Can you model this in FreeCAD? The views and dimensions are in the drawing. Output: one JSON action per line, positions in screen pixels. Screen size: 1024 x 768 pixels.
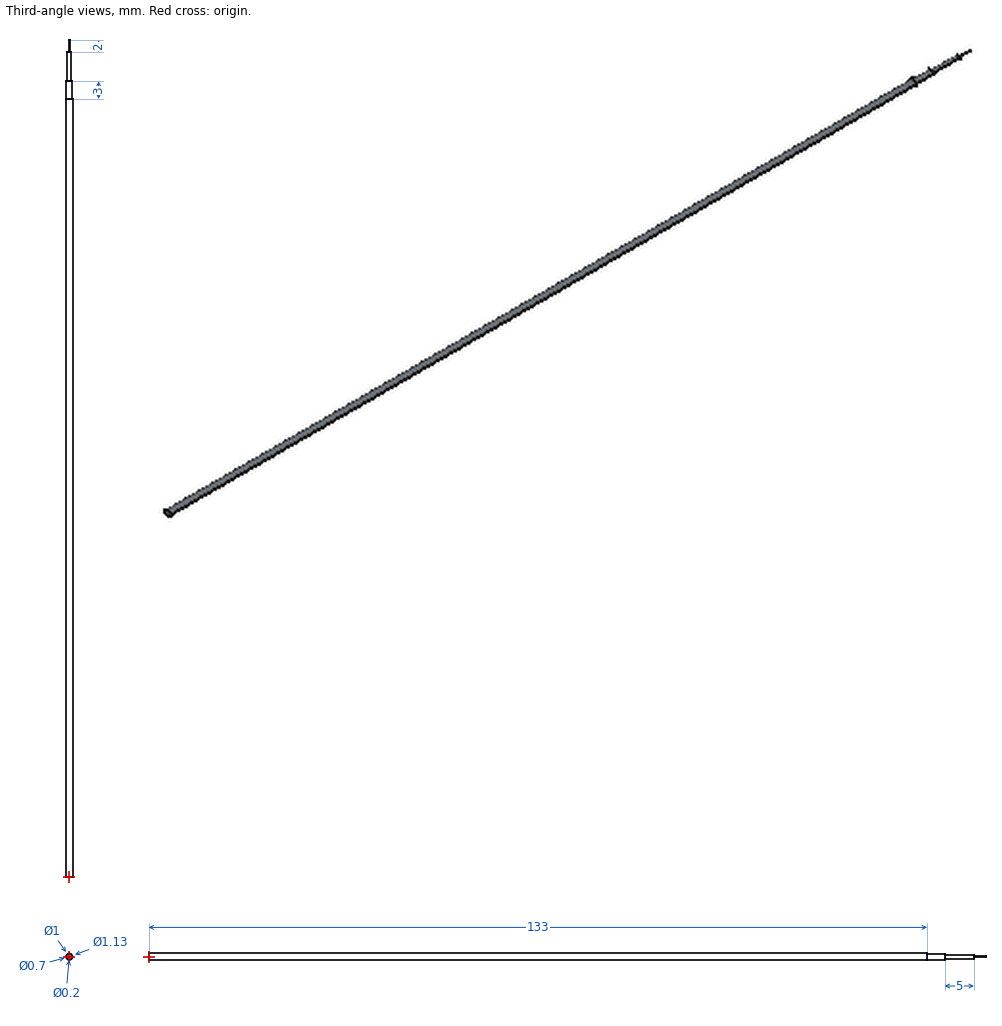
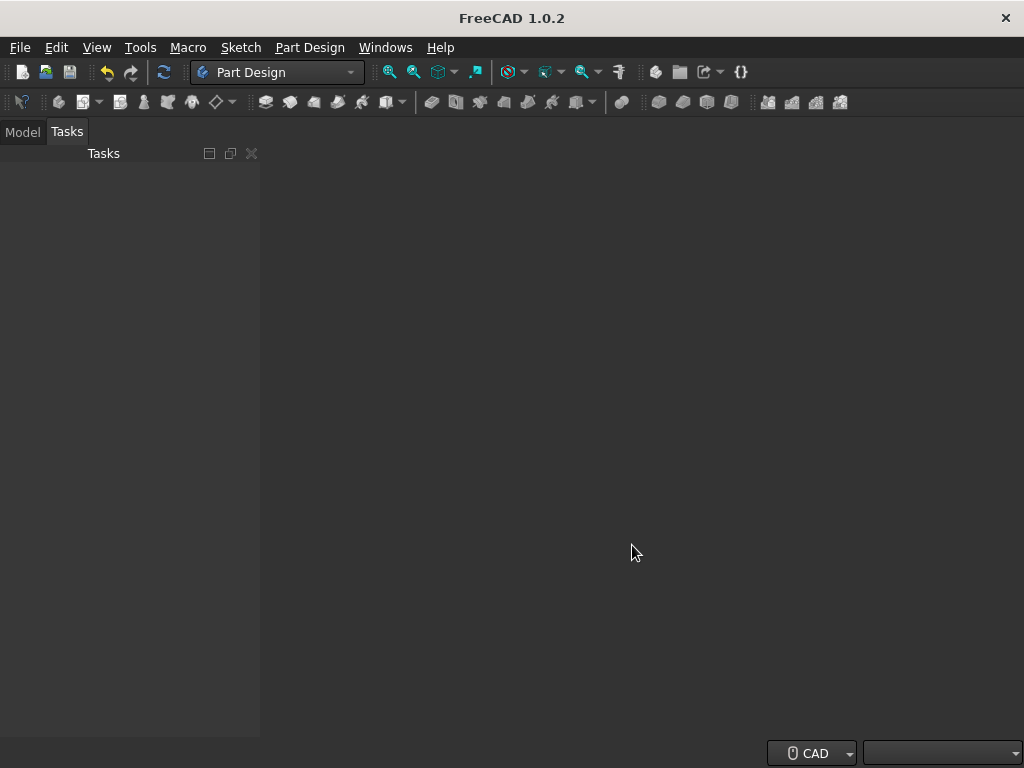
{"action": "left_click", "coordinate": [22, 72]}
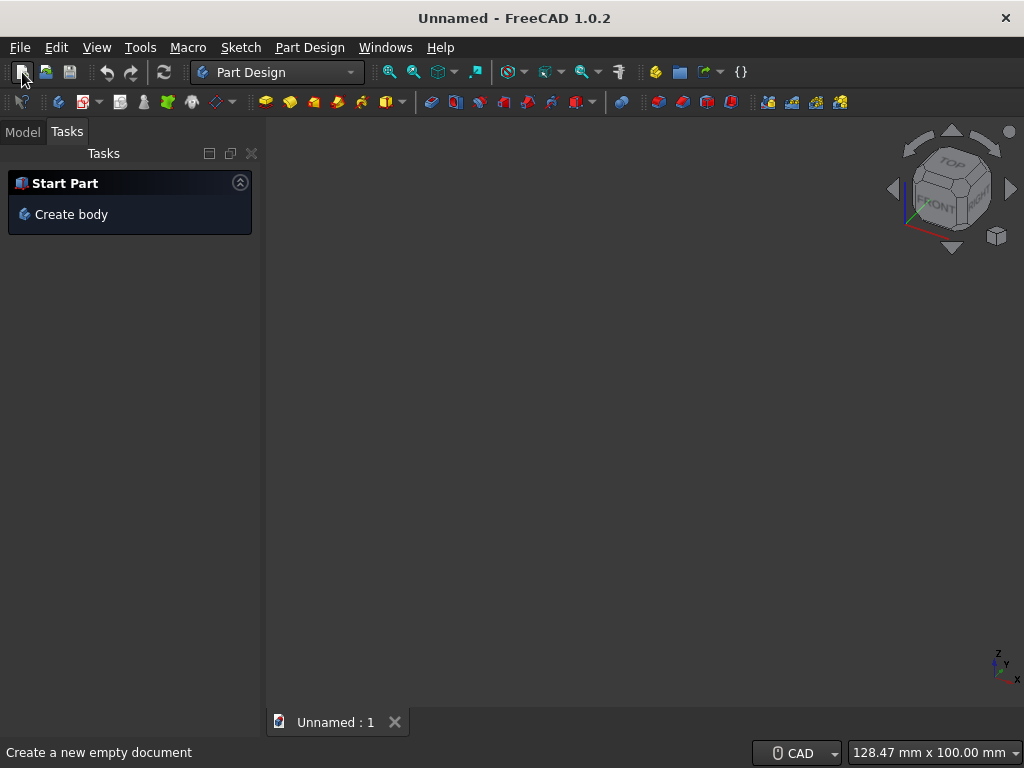
{"action": "left_click", "coordinate": [84, 102]}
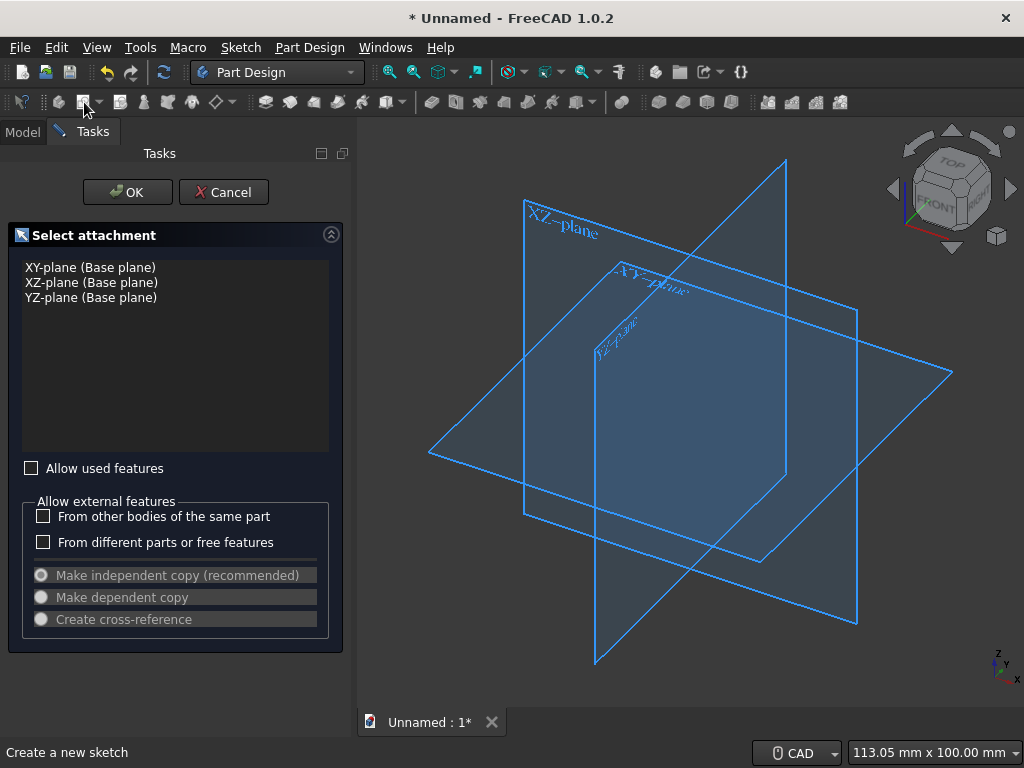
{"action": "left_click", "coordinate": [82, 282]}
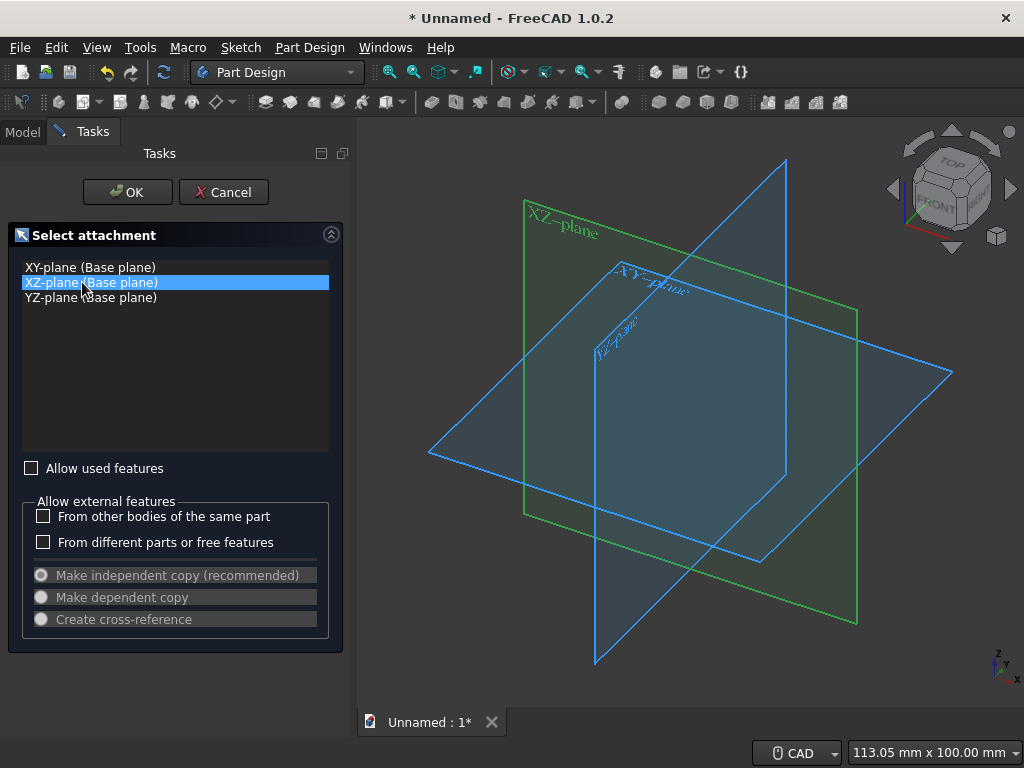
{"action": "left_click", "coordinate": [128, 192]}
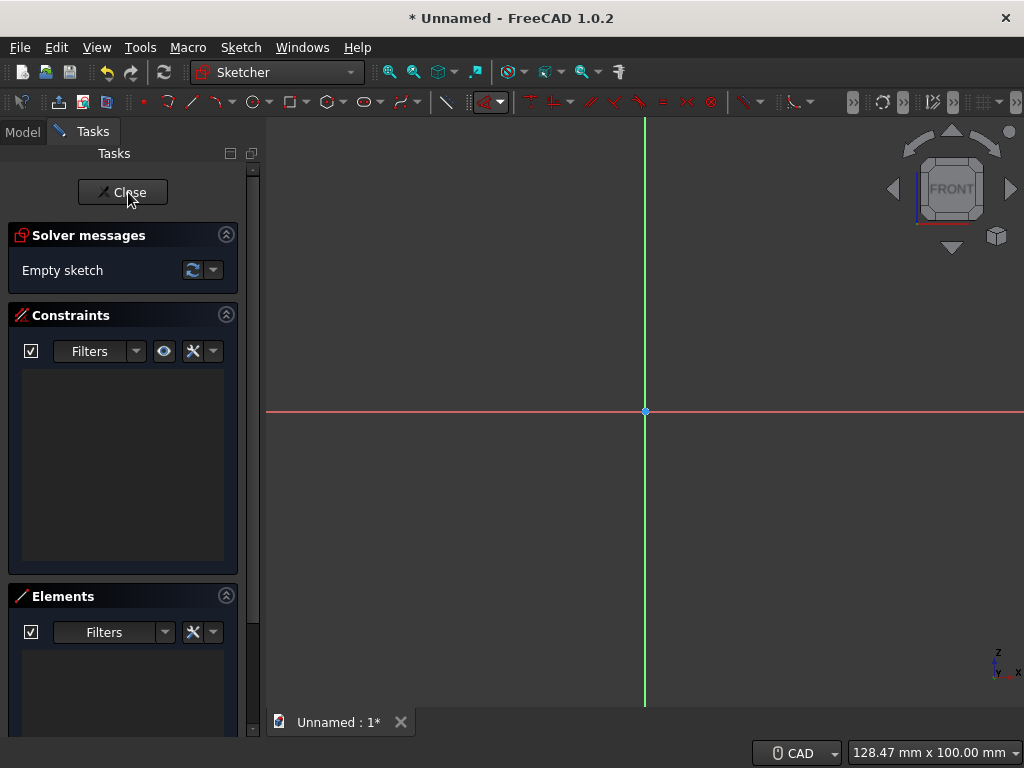
{"action": "scroll", "coordinate": [649, 412], "scroll_direction": "up", "scroll_amount": 15}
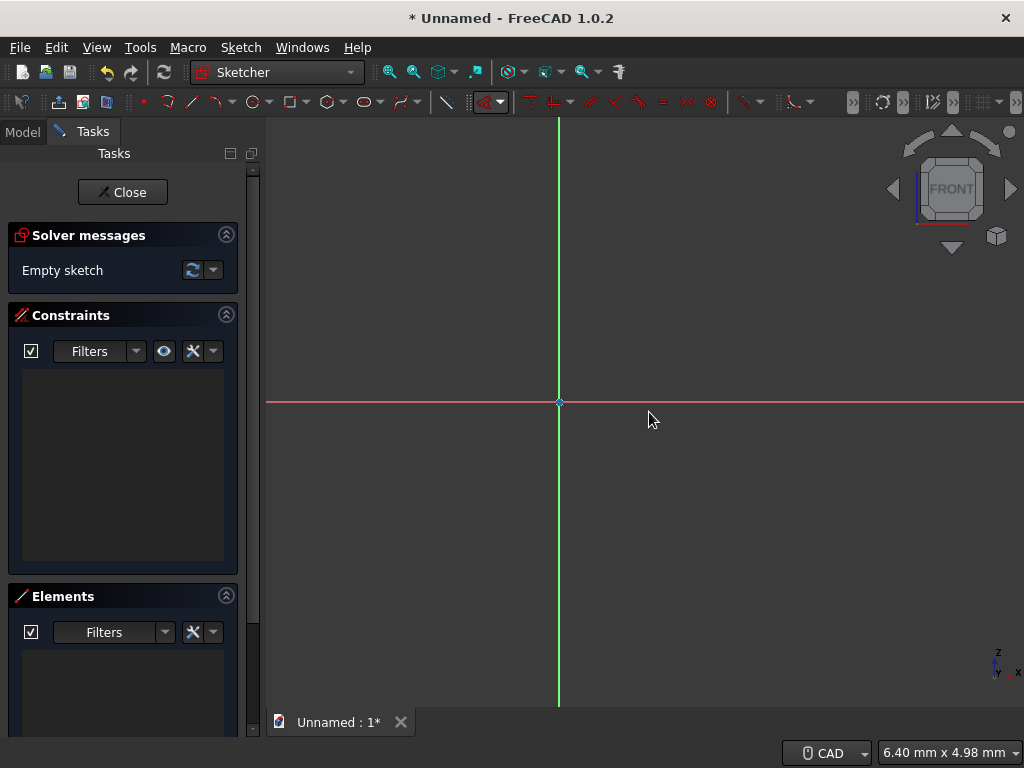
{"action": "scroll", "coordinate": [549, 397], "scroll_direction": "up", "scroll_amount": 5}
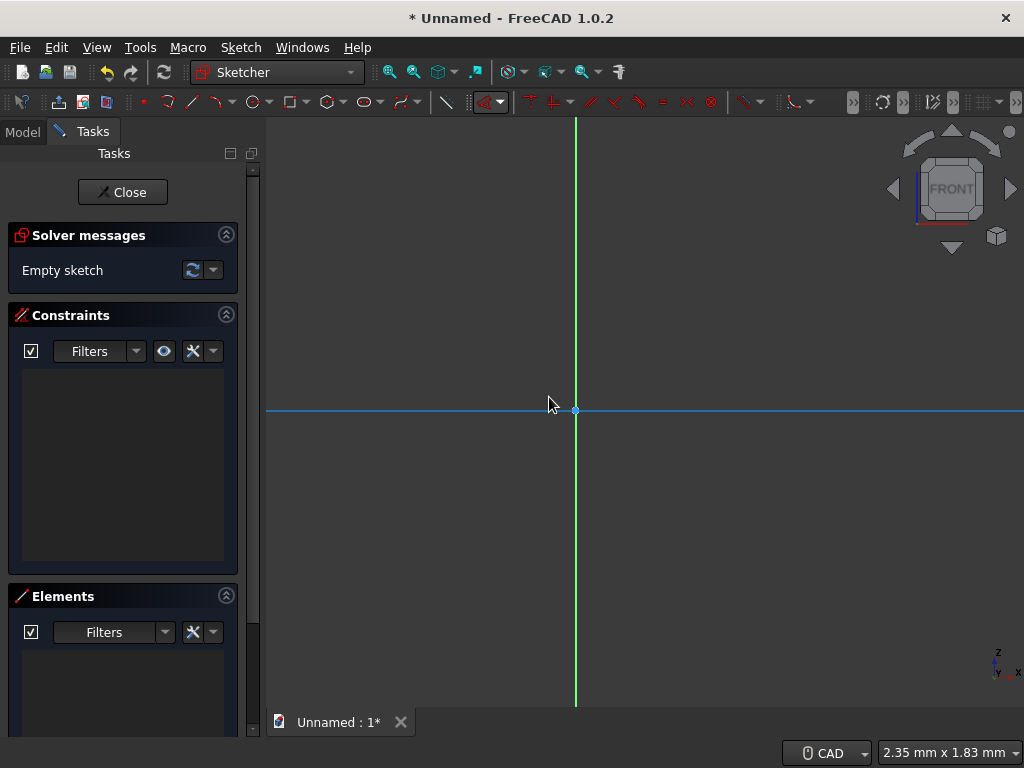
{"action": "left_click", "coordinate": [254, 102]}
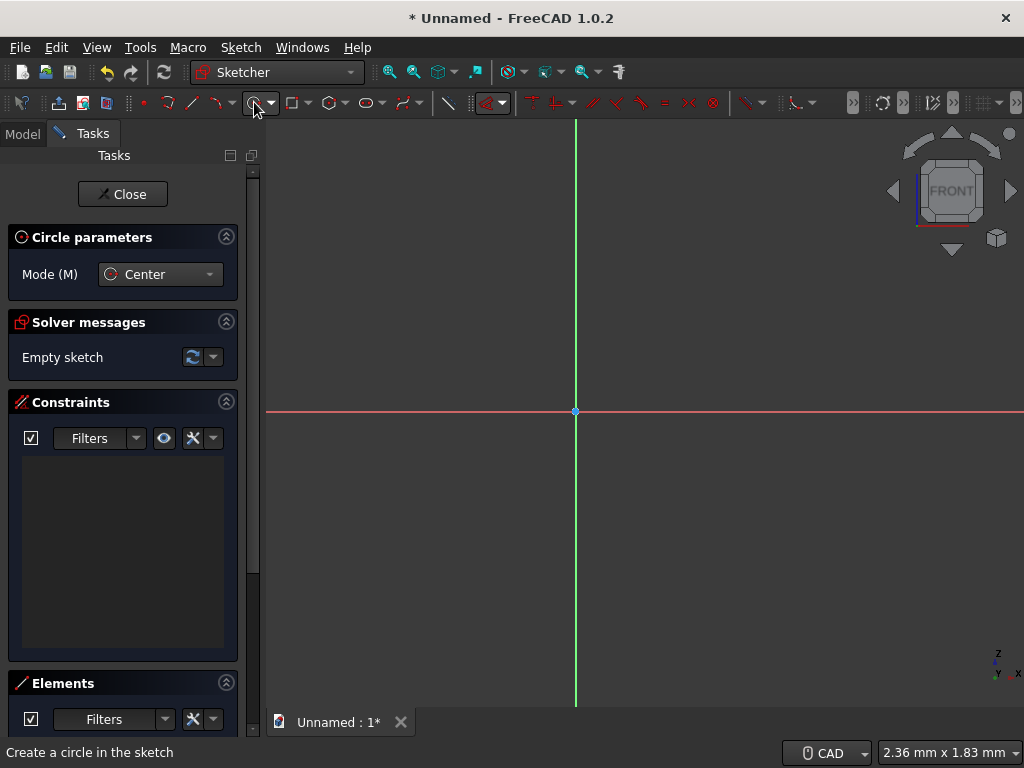
{"action": "left_click", "coordinate": [576, 412]}
{"action": "left_click", "coordinate": [704, 284]}
{"action": "key", "text": "Escape"}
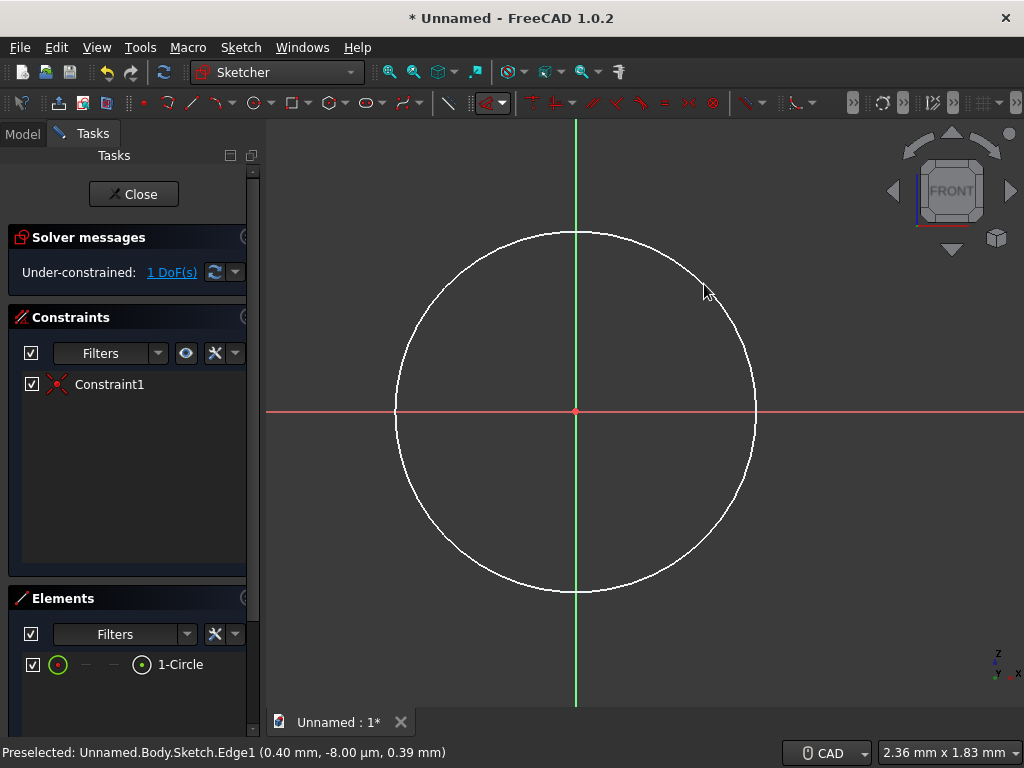
{"action": "left_click", "coordinate": [703, 284]}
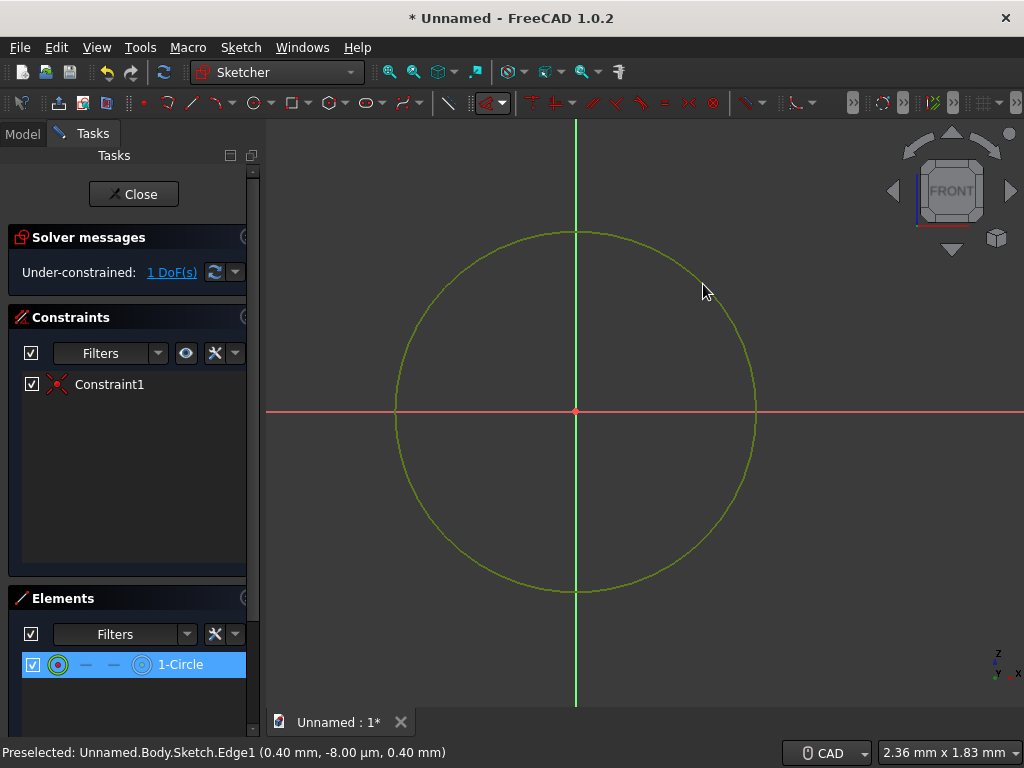
{"action": "key", "text": "k o"}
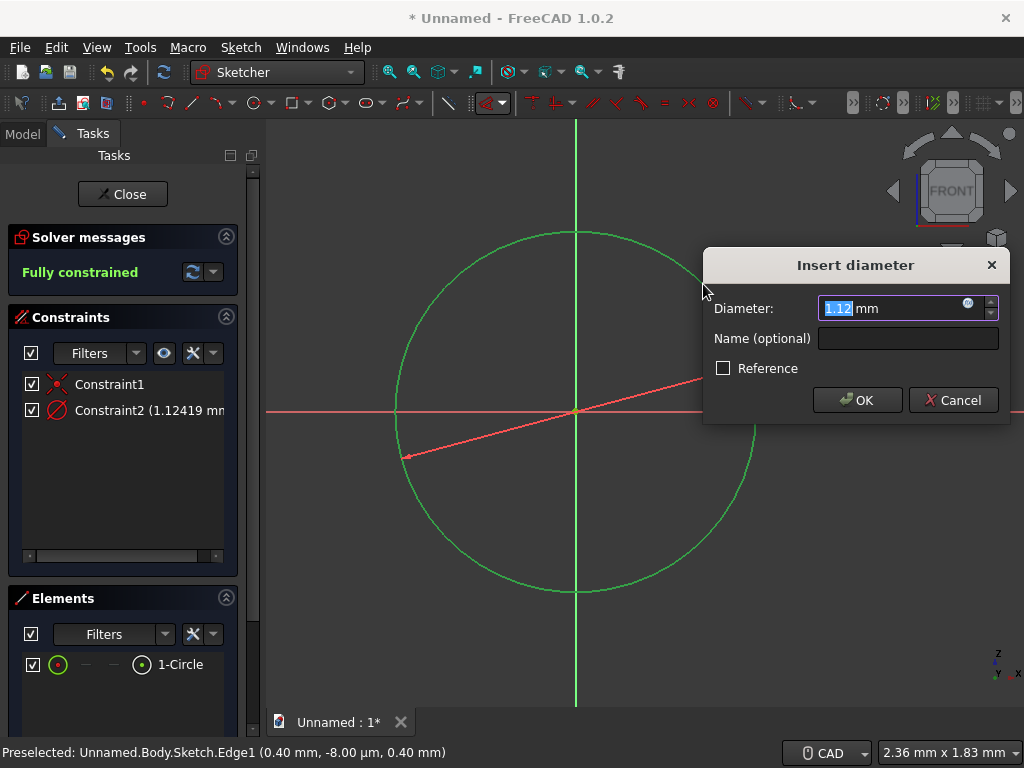
{"action": "type", "text": "1.13"}
{"action": "key", "text": "Return"}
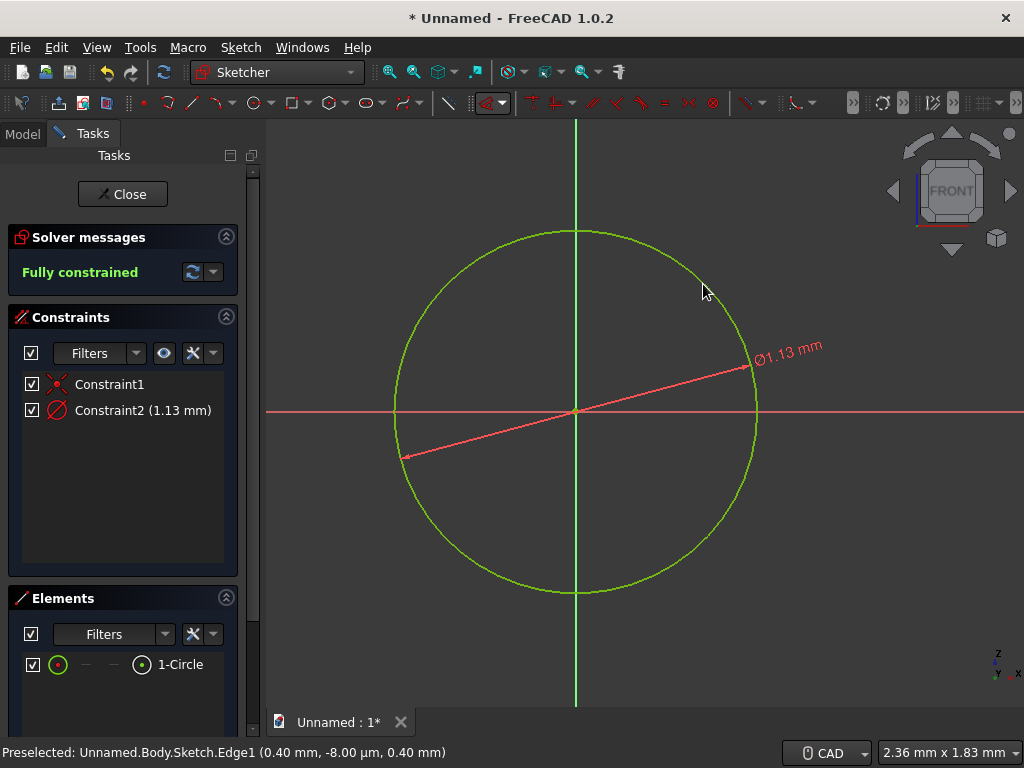
{"action": "left_click", "coordinate": [123, 194]}